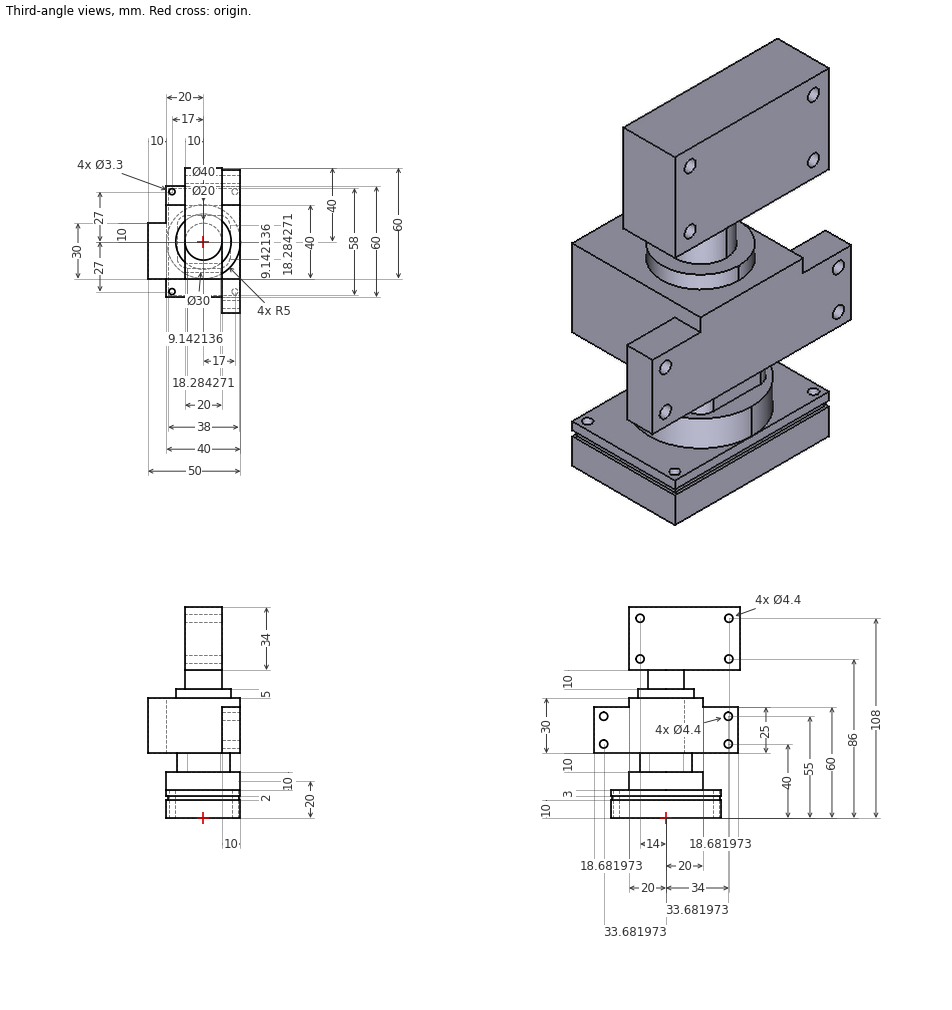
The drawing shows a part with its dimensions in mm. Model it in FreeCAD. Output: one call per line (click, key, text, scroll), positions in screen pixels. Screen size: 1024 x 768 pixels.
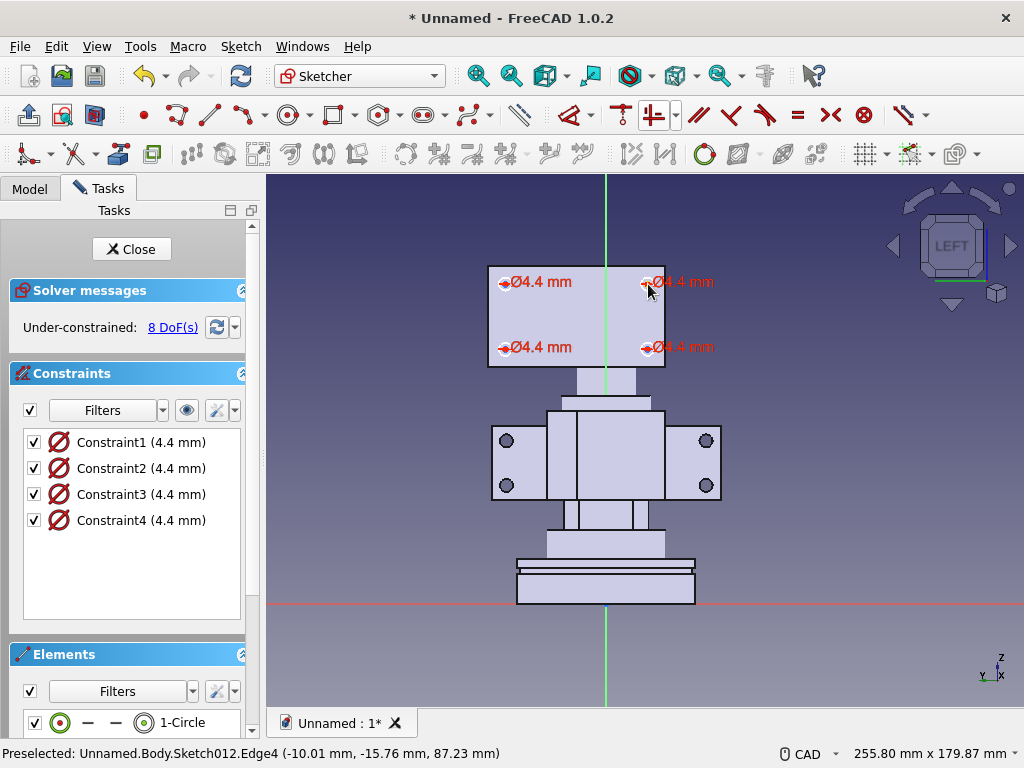
click(505, 284)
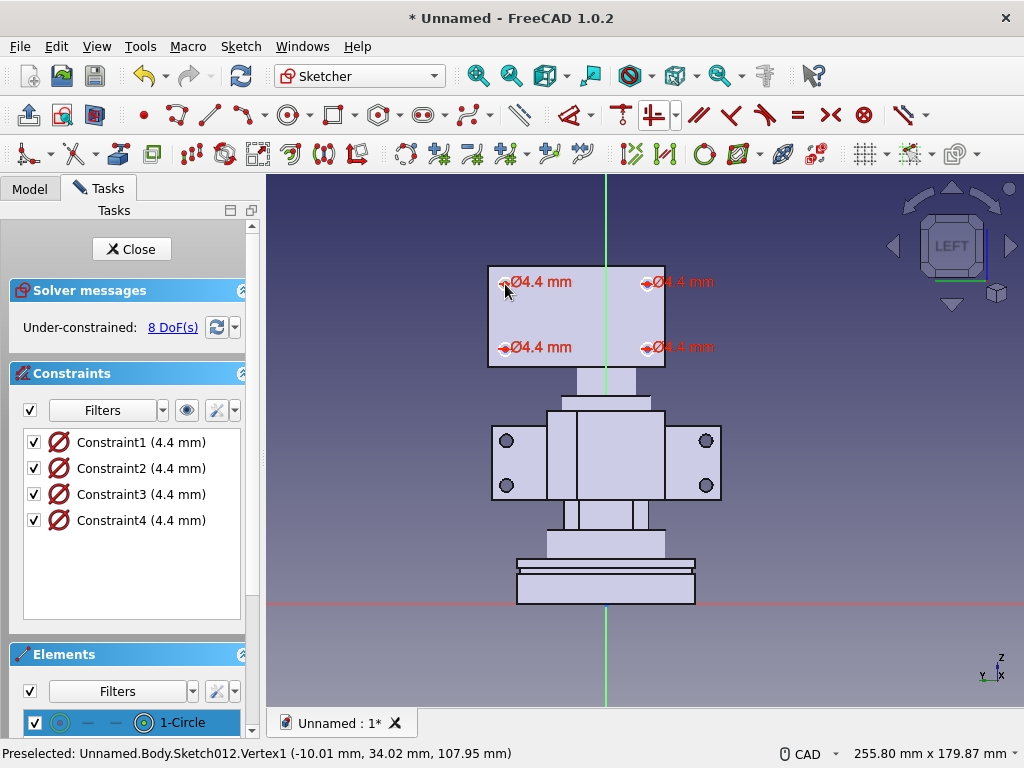
click(505, 349)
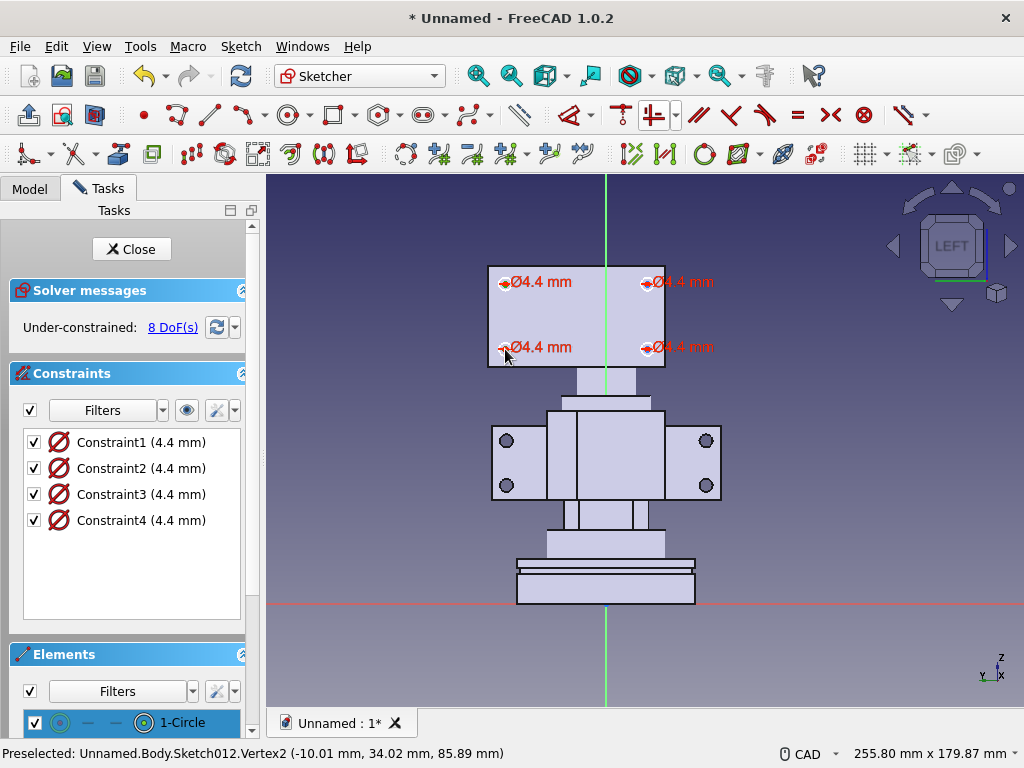
key(v)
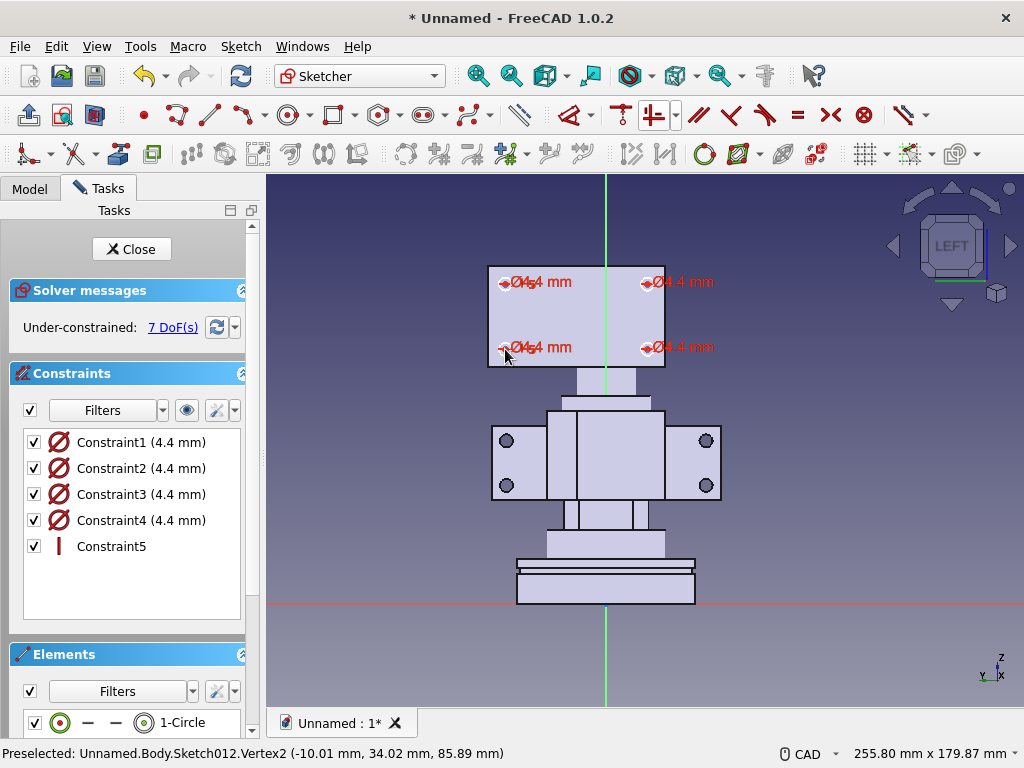
click(505, 284)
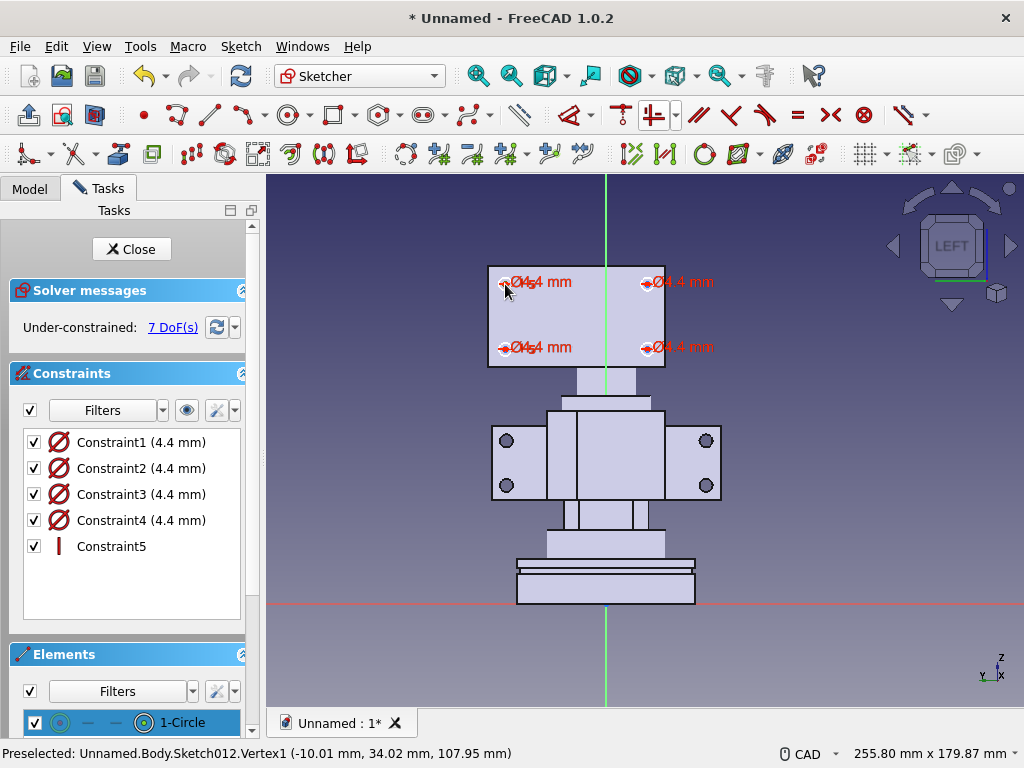
click(648, 284)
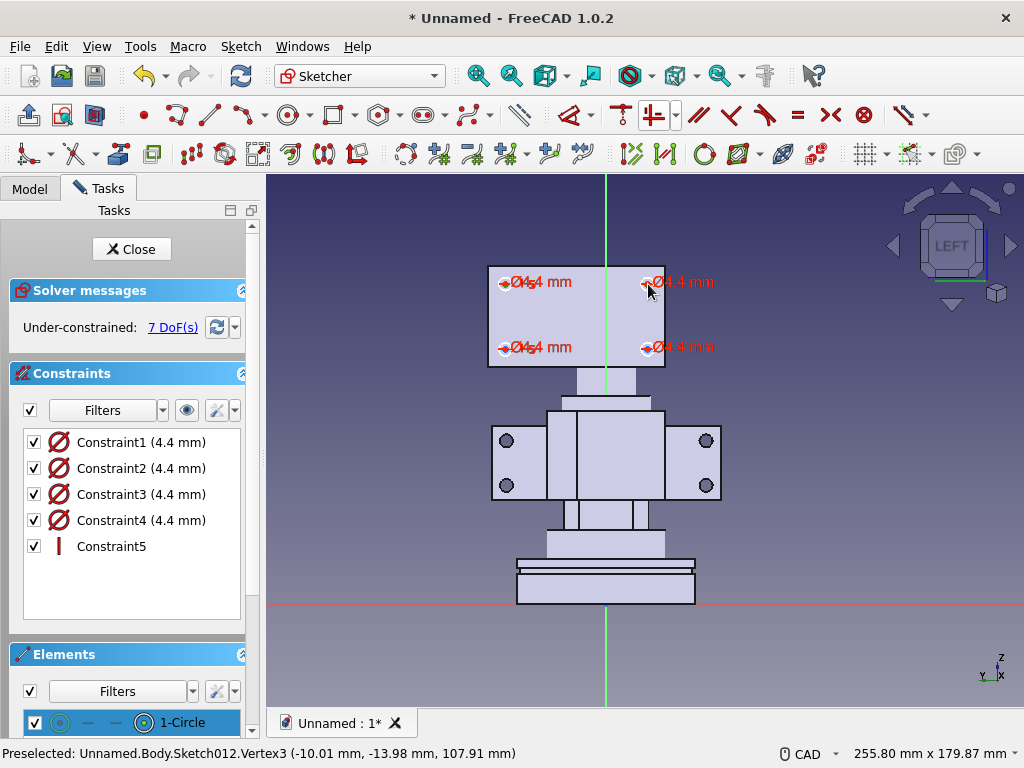
key(h)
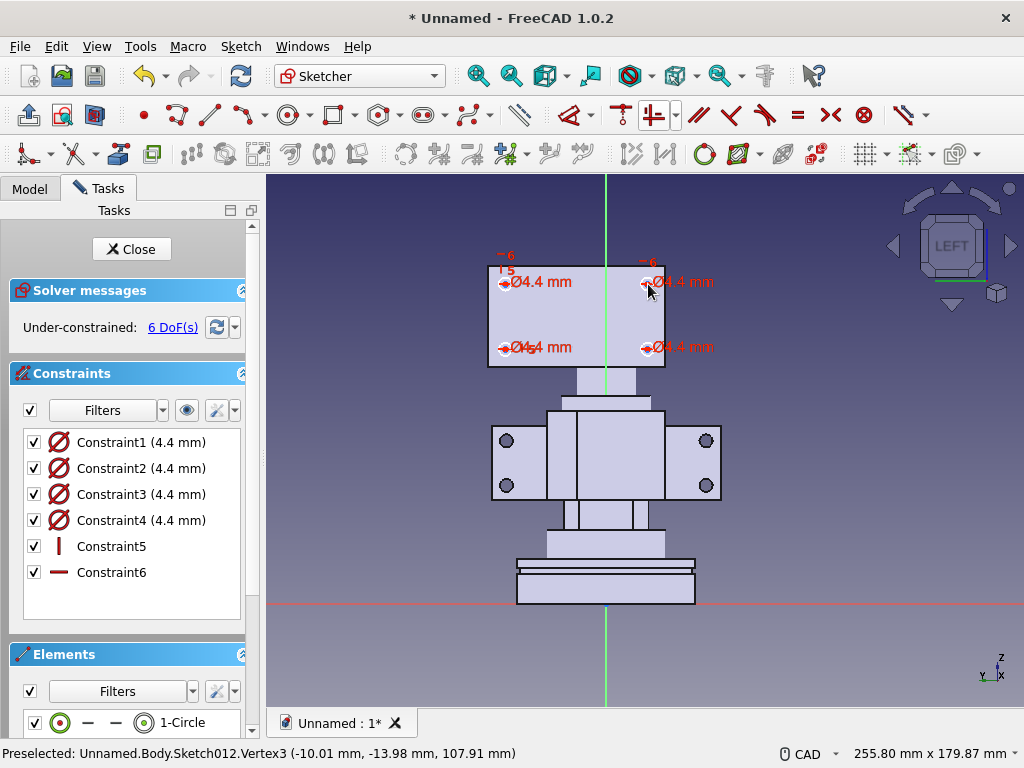
click(648, 284)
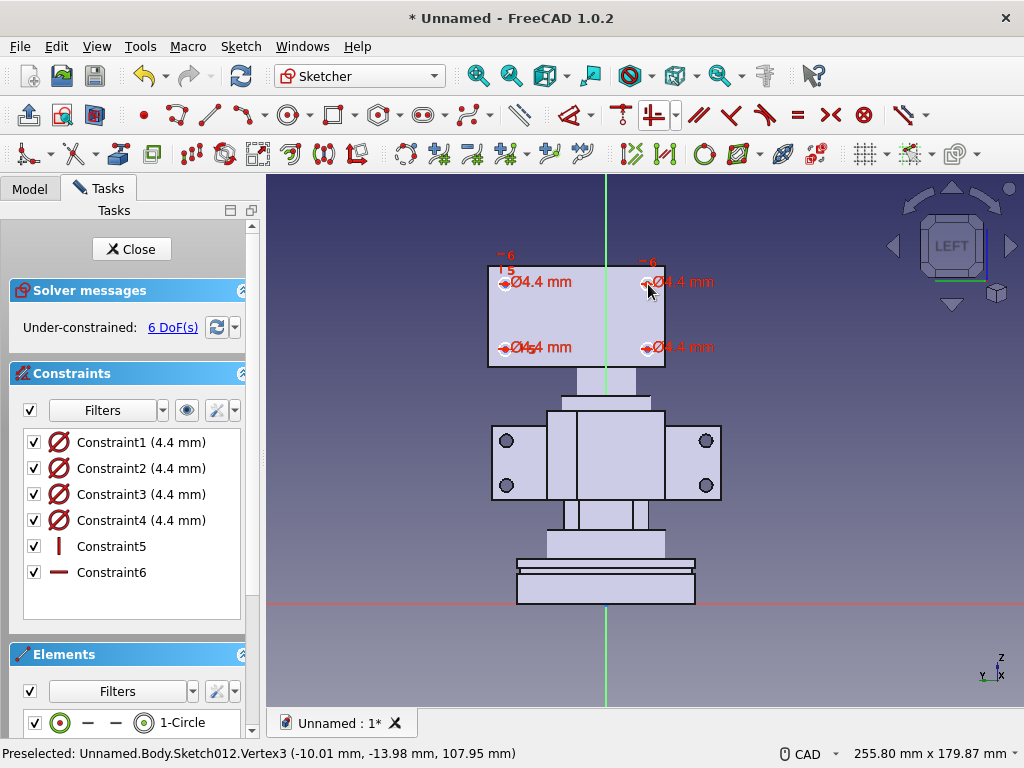
click(648, 349)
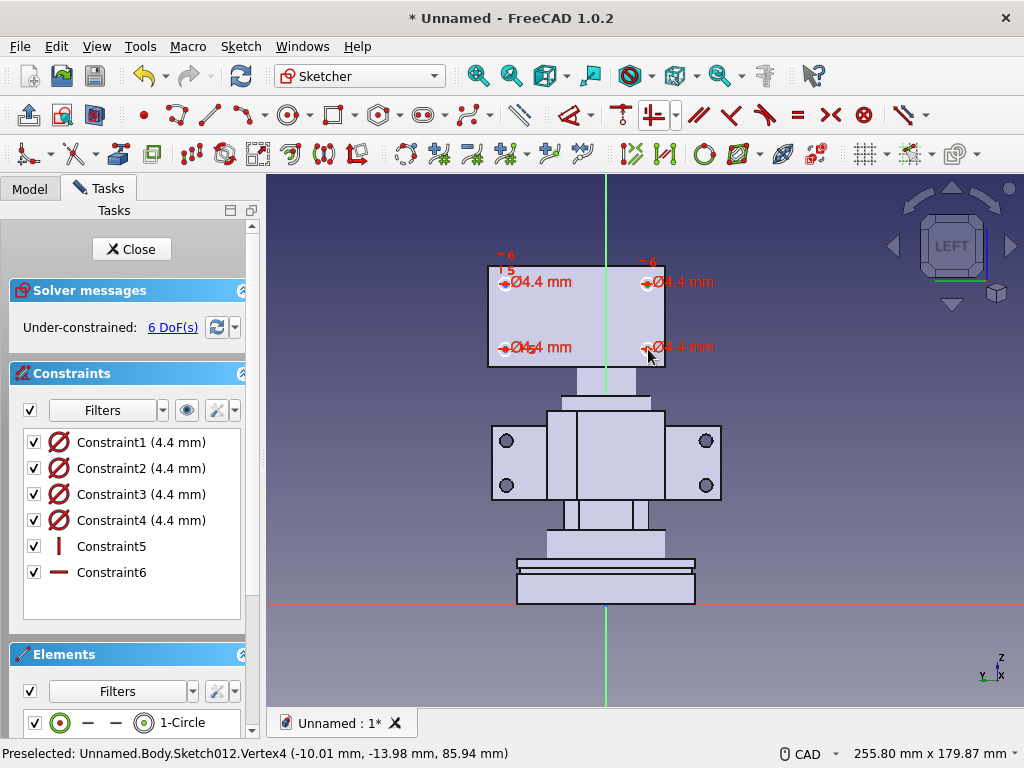
click(676, 116)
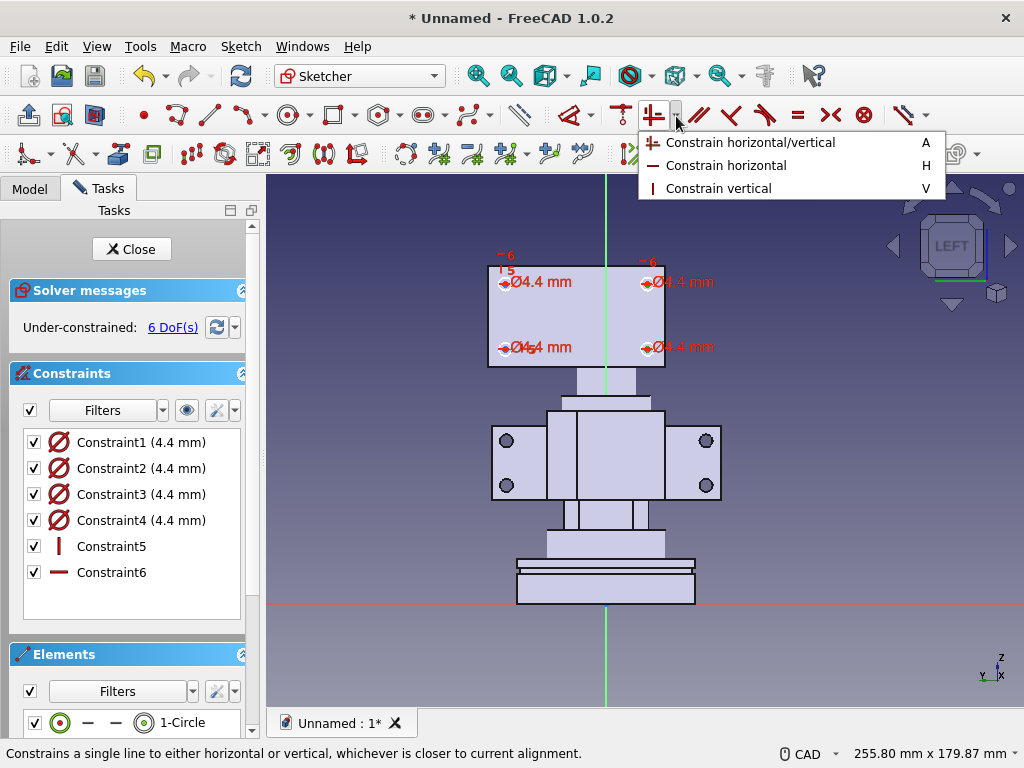
click(792, 188)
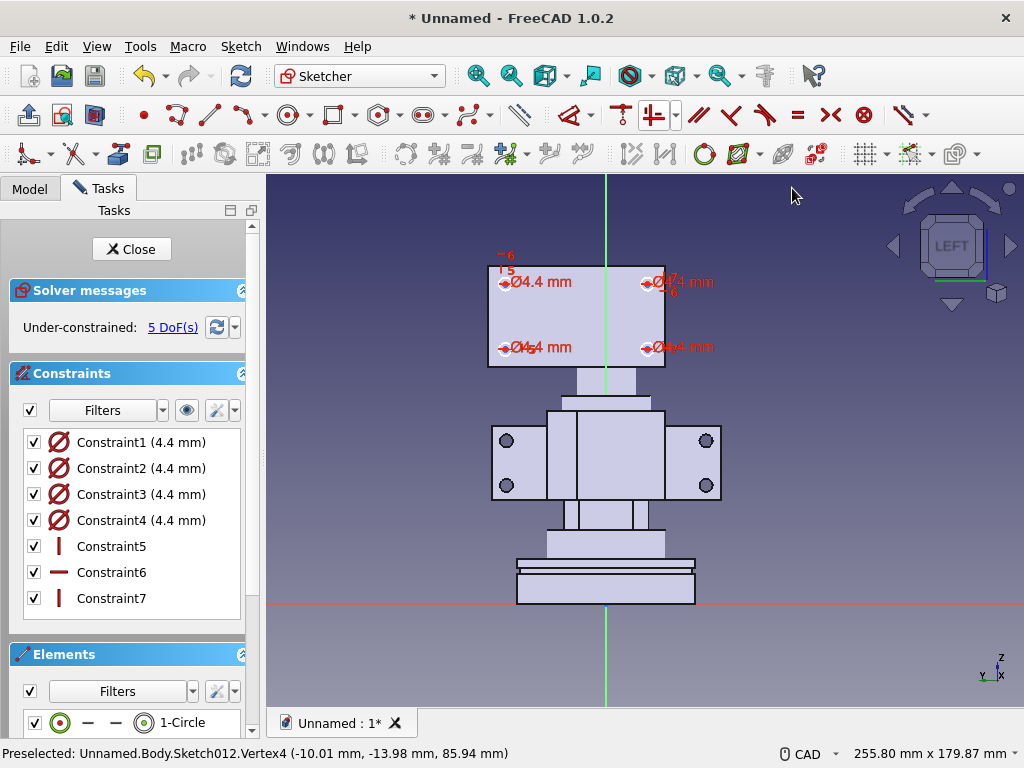
click(505, 349)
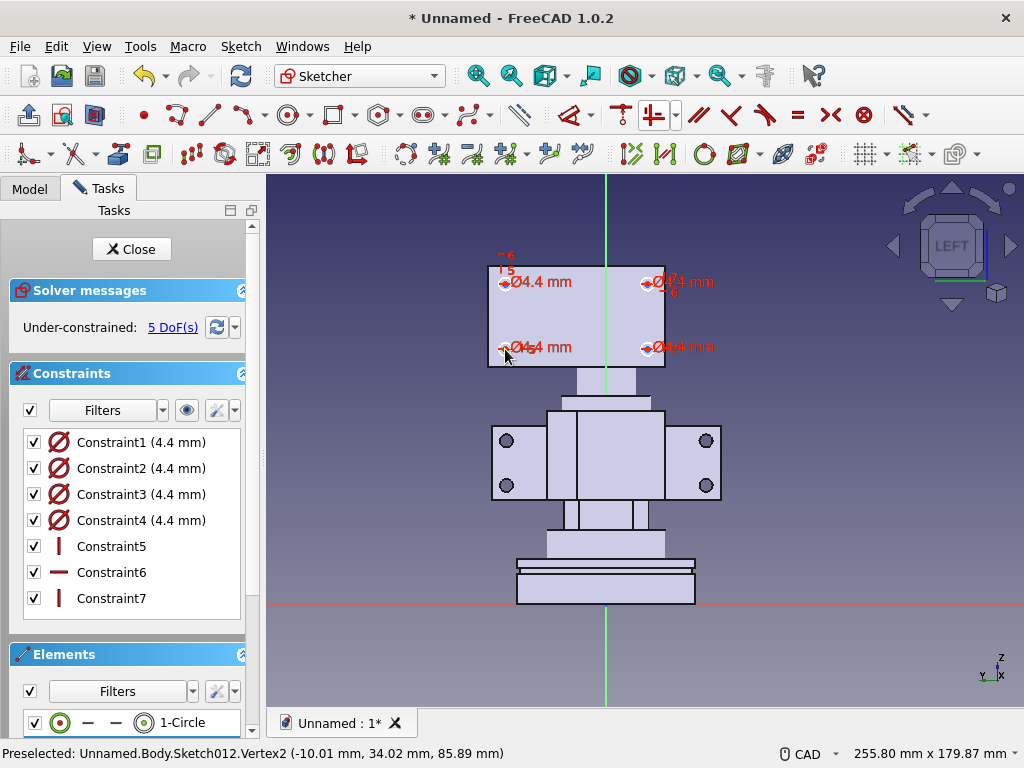
click(648, 349)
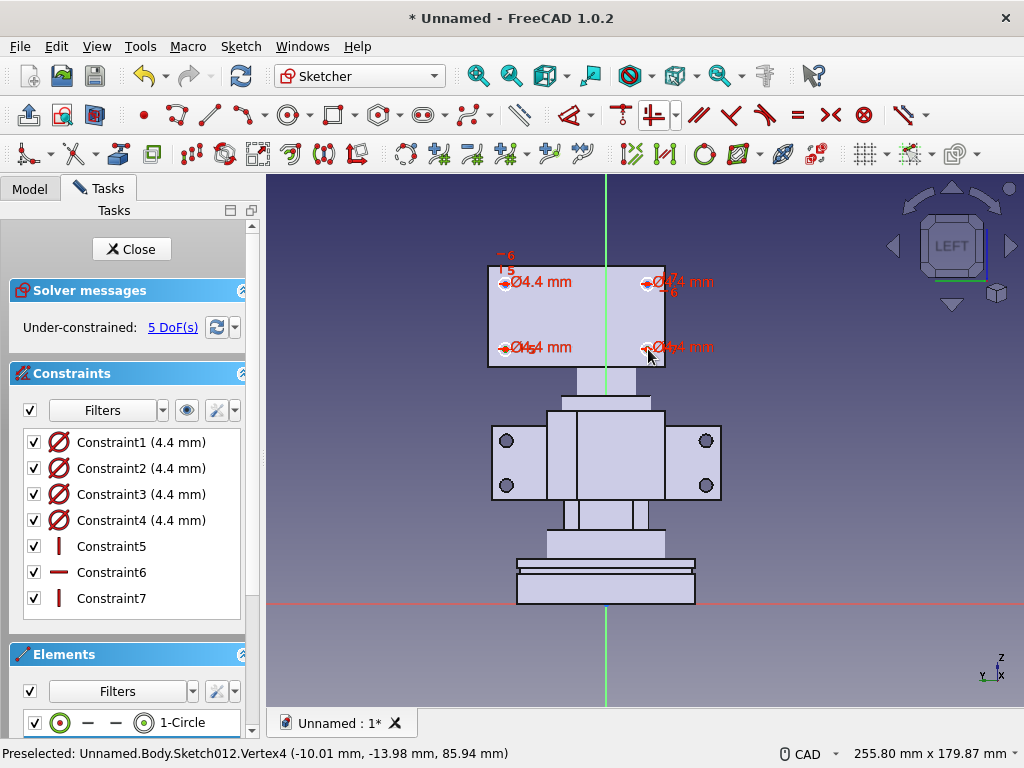
key(h)